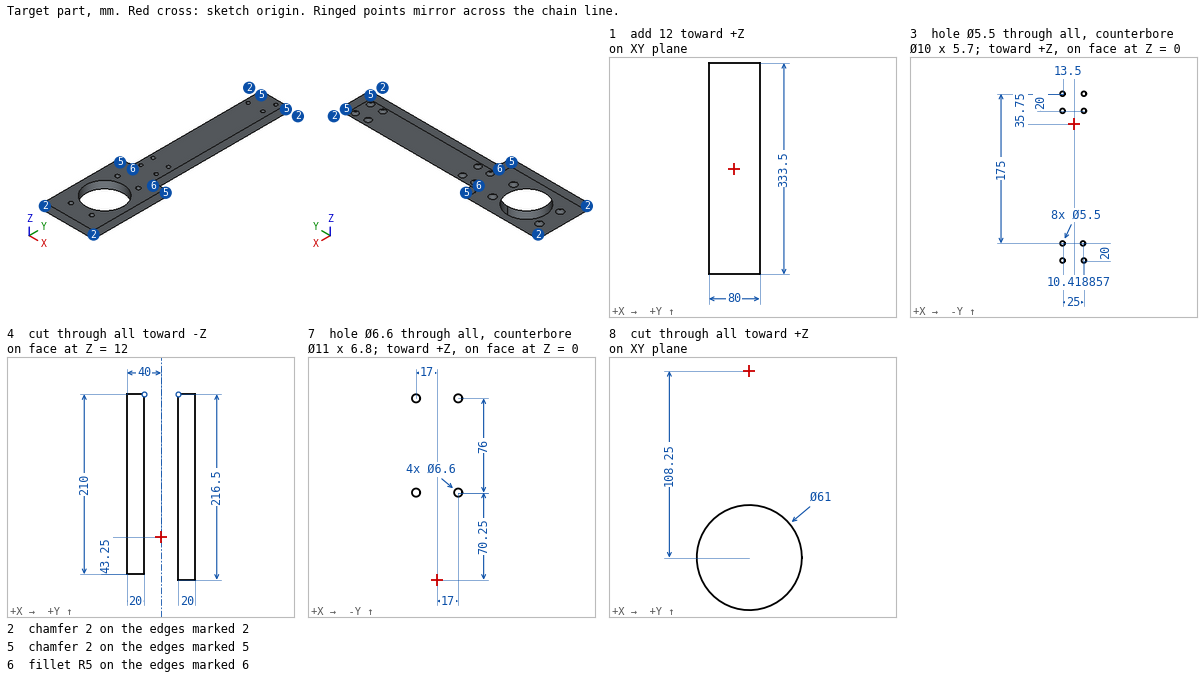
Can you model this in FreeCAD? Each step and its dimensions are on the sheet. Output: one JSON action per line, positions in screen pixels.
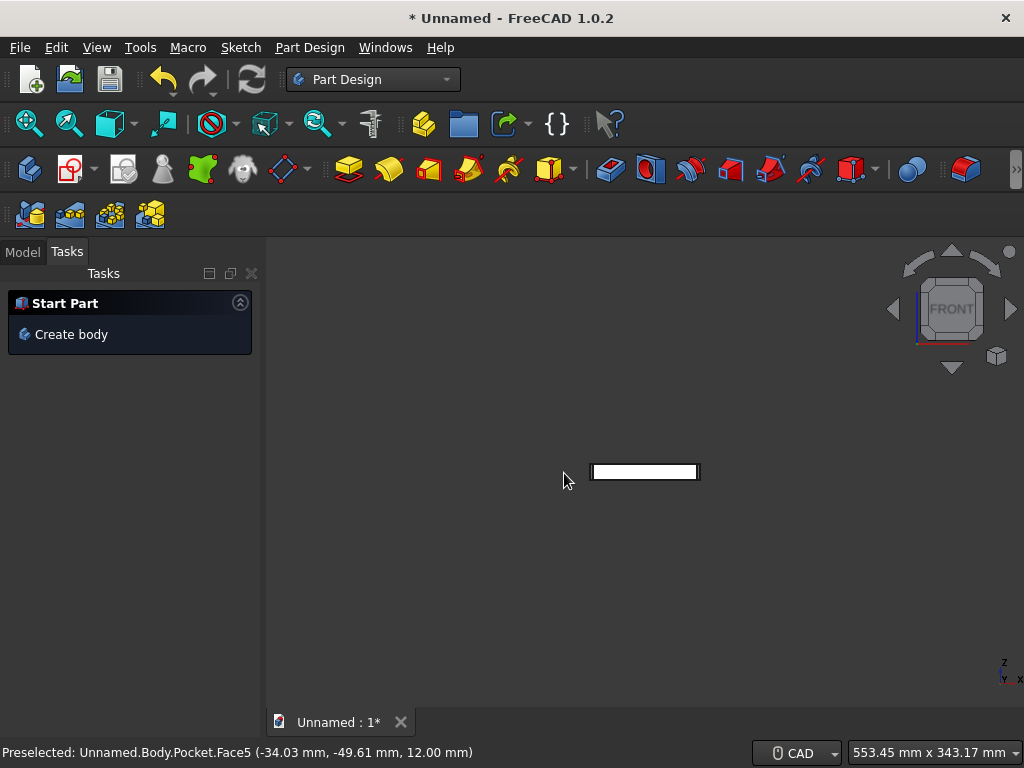
{"action": "key", "text": "v f"}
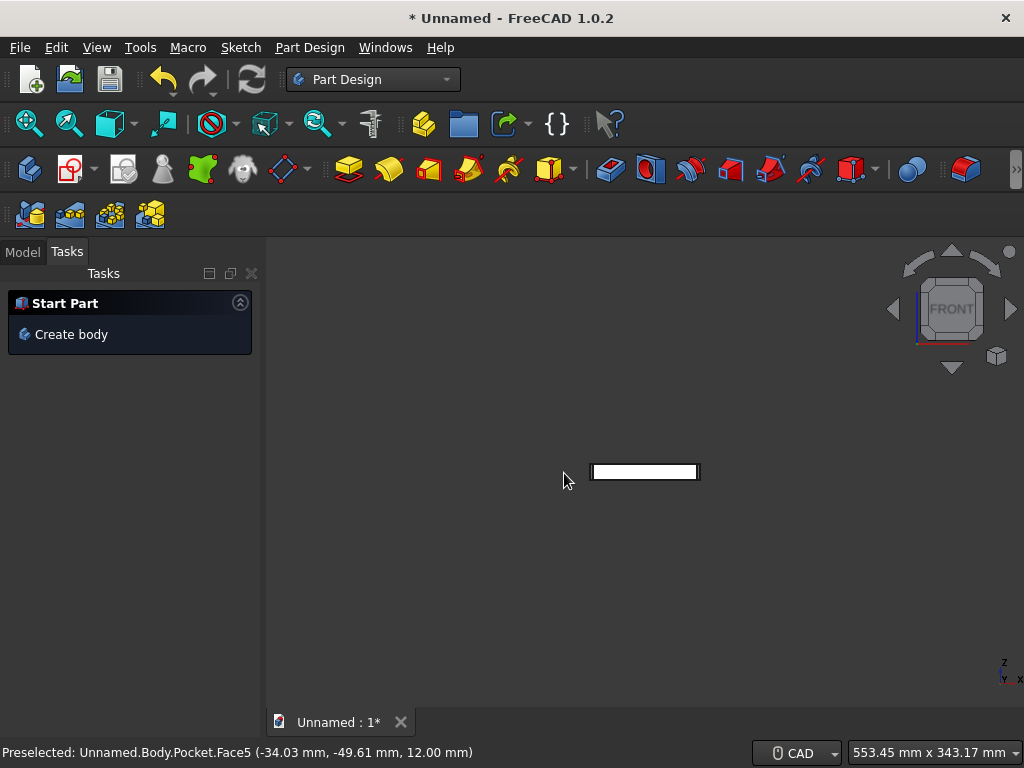
{"action": "scroll", "coordinate": [590, 471], "scroll_direction": "up", "scroll_amount": 5}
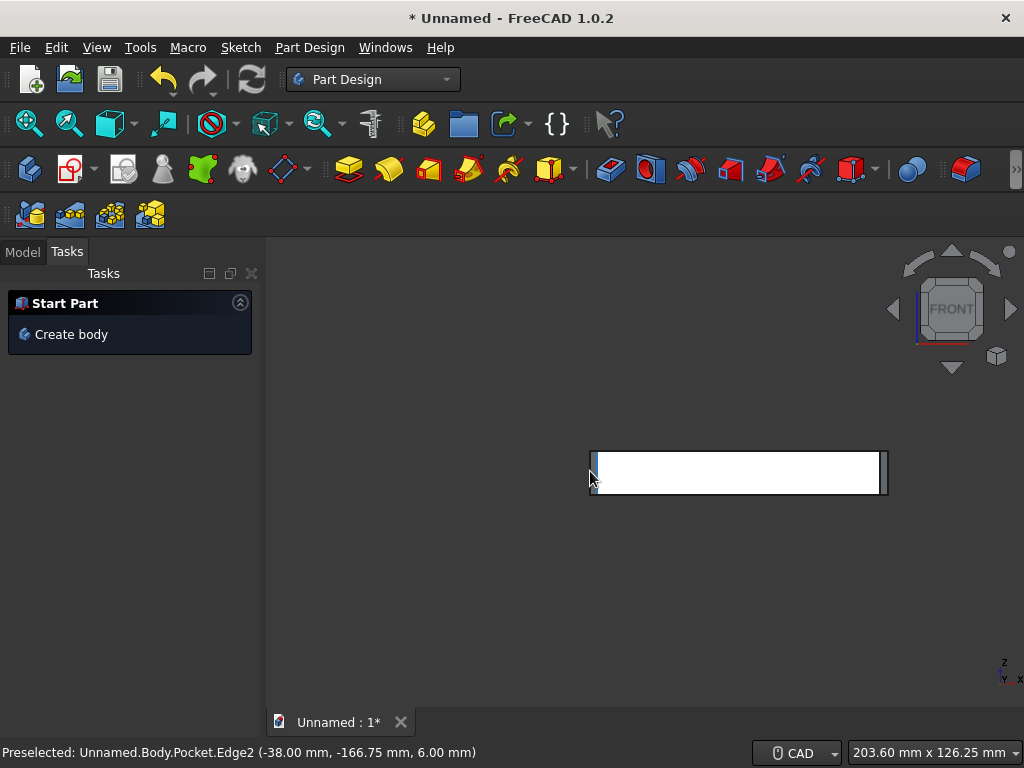
{"action": "key", "text": "v f"}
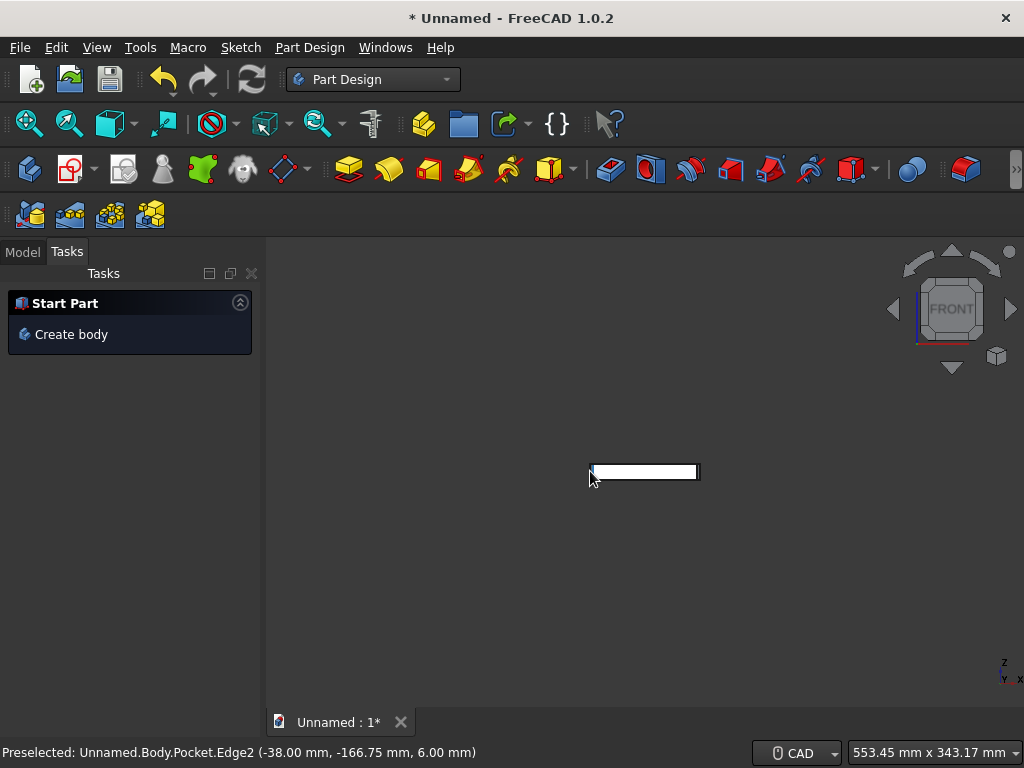
{"action": "key", "text": "3"}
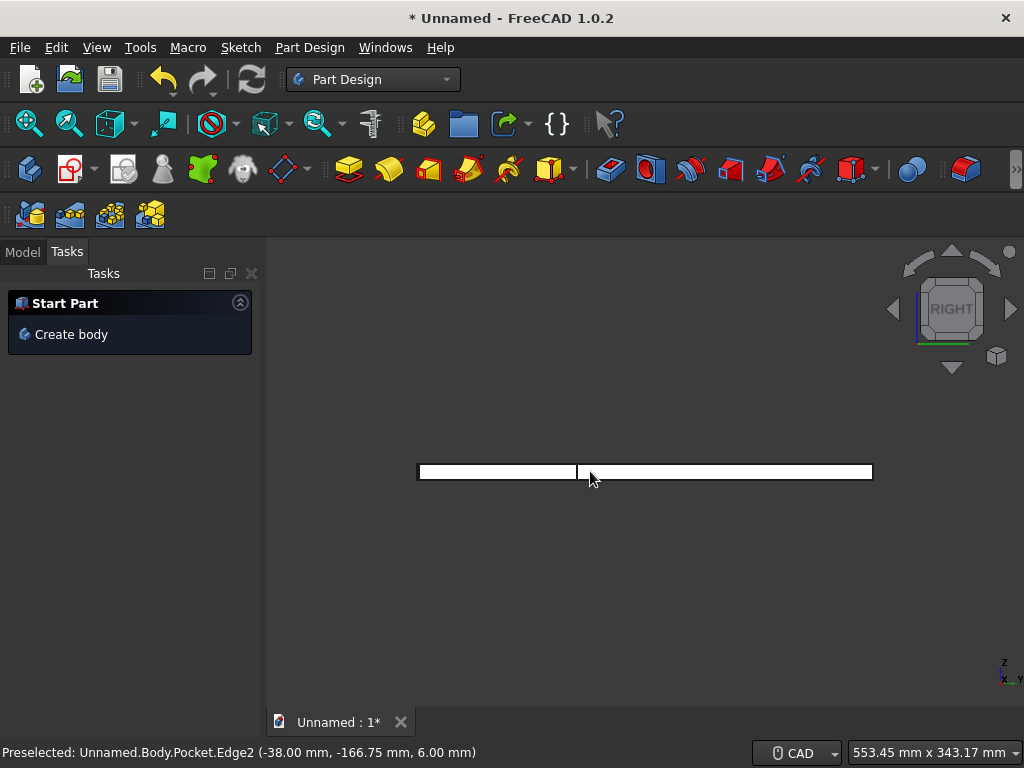
{"action": "left_click", "coordinate": [577, 471]}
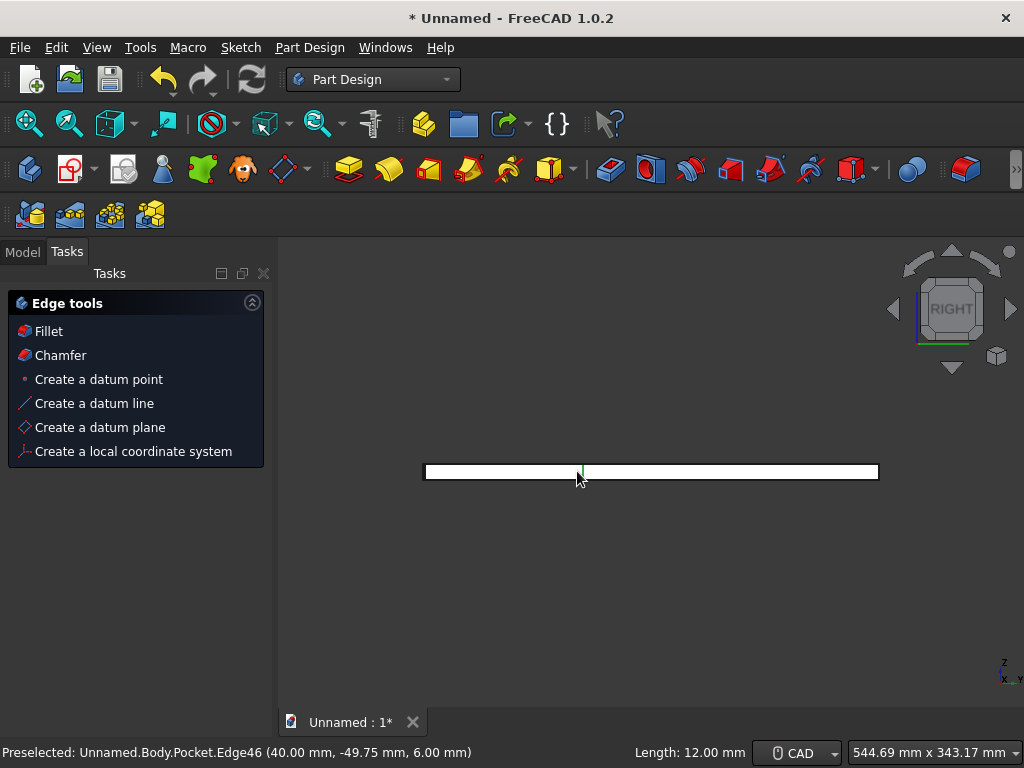
{"action": "left_click", "coordinate": [879, 471], "text": "ctrl"}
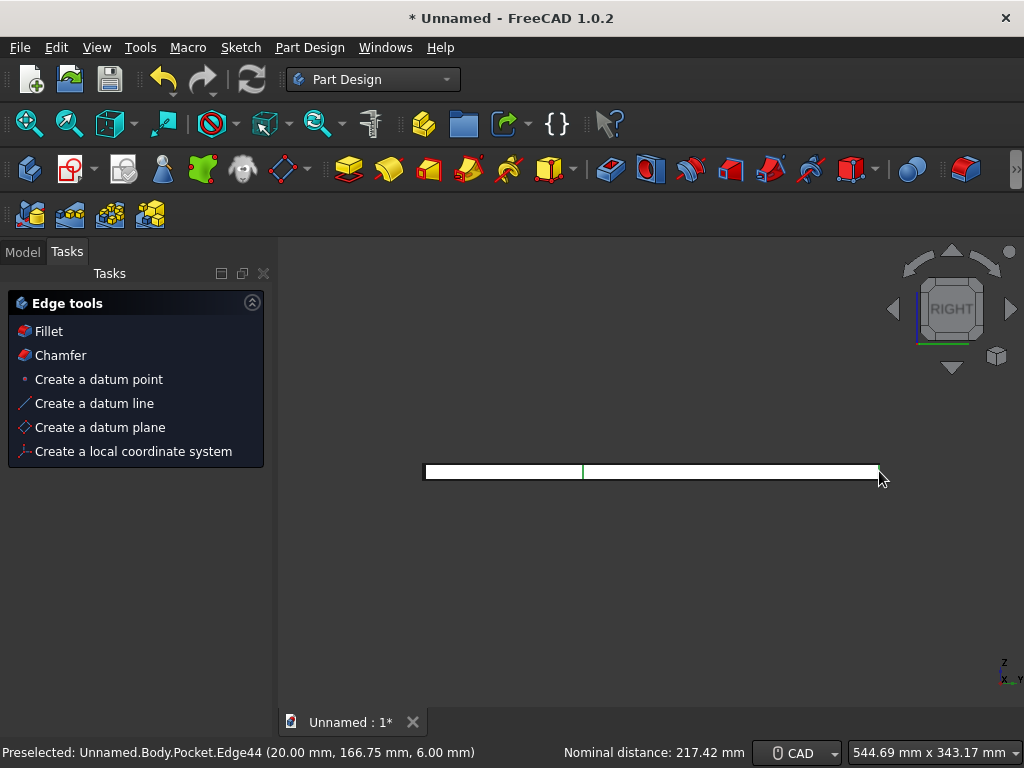
{"action": "scroll", "coordinate": [592, 471], "scroll_direction": "up", "scroll_amount": 5}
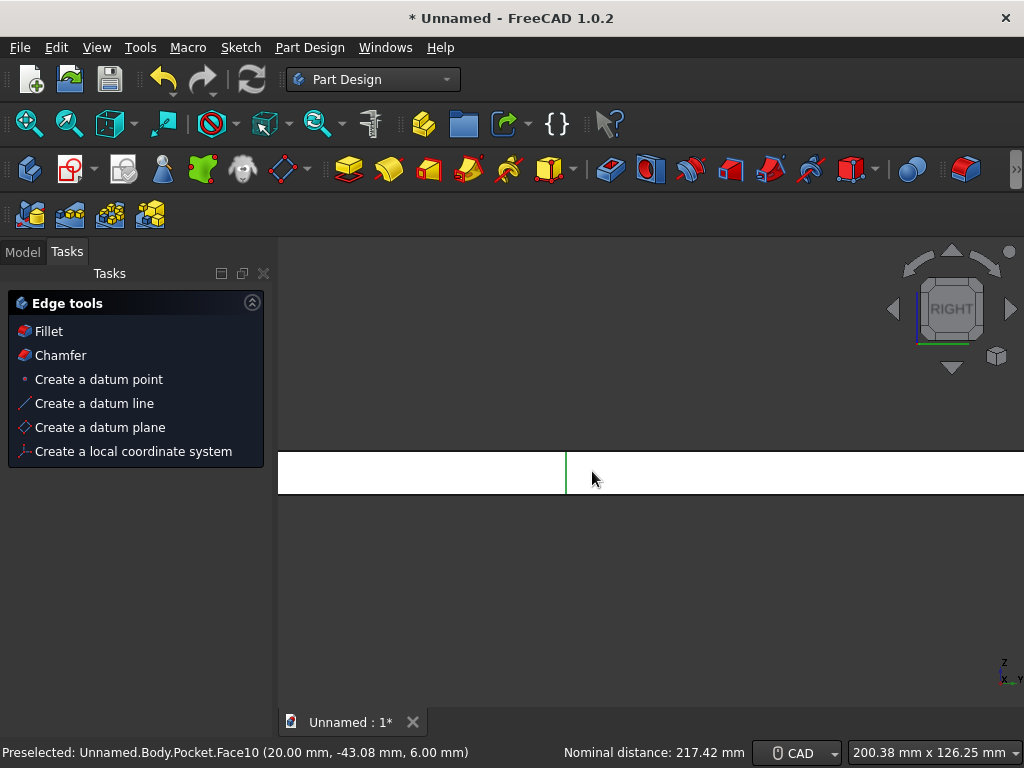
{"action": "left_click", "coordinate": [30, 124]}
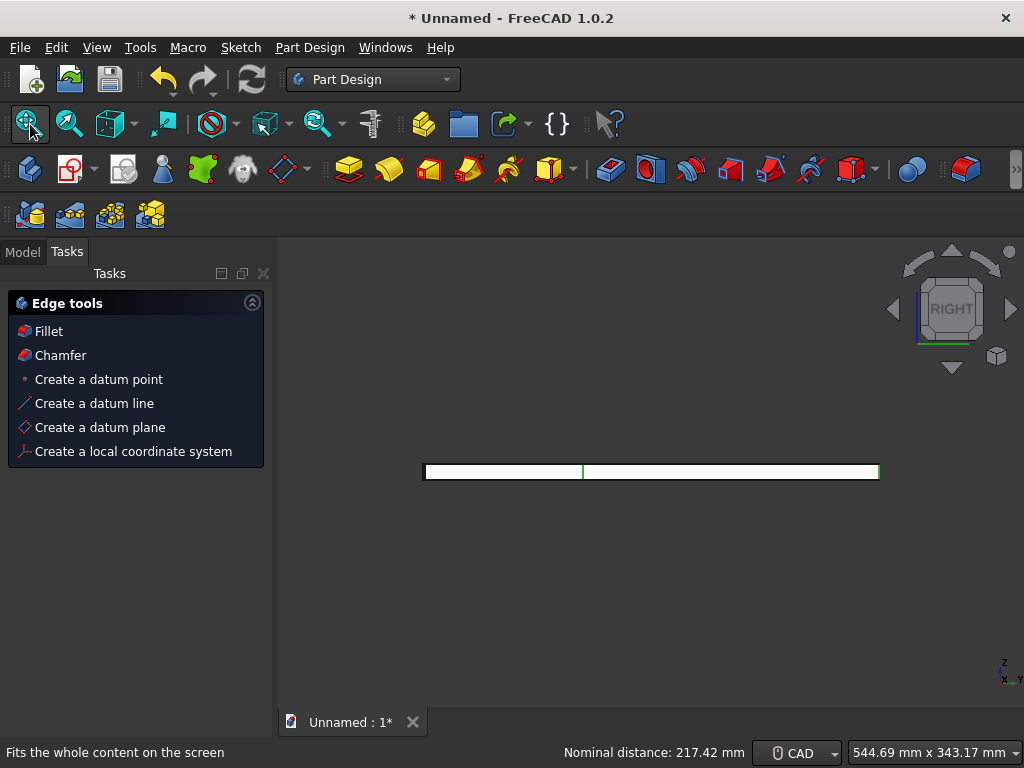
{"action": "key", "text": "5"}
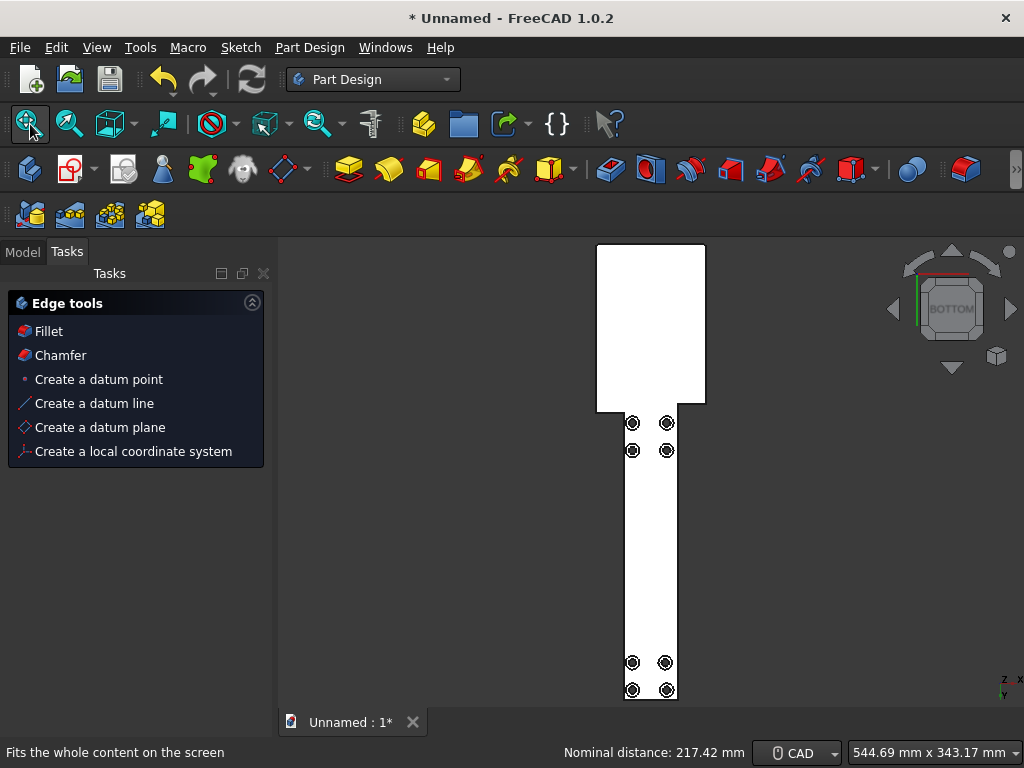
{"action": "scroll", "coordinate": [596, 412], "scroll_direction": "up", "scroll_amount": 5}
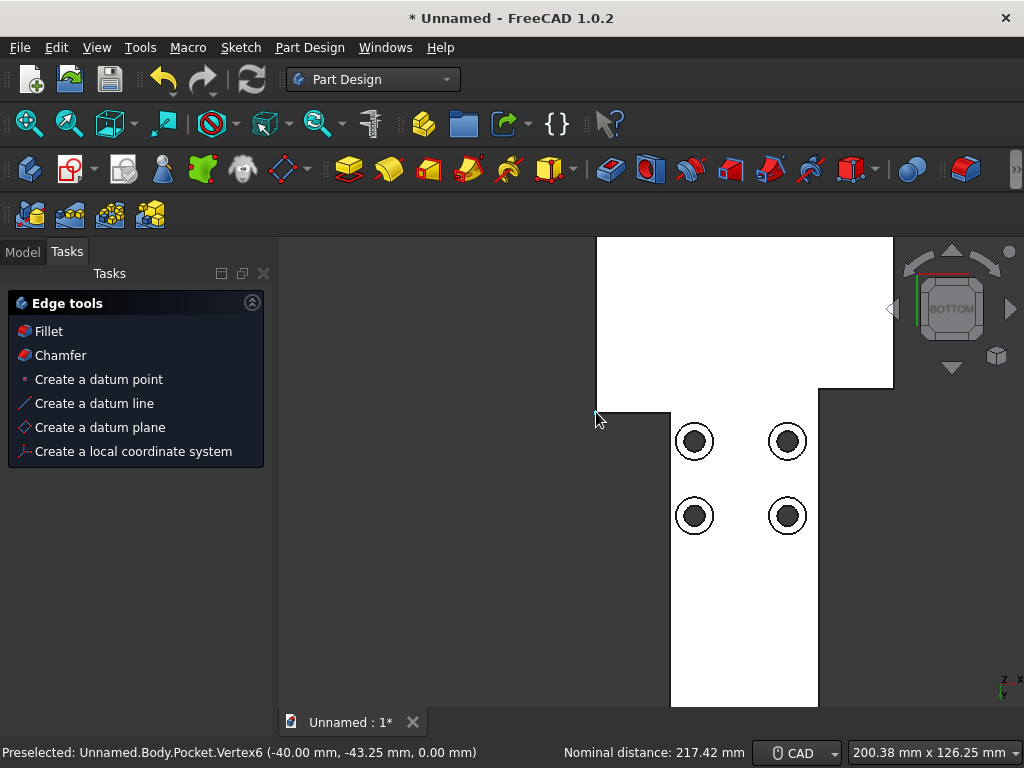
{"action": "key", "text": "v f"}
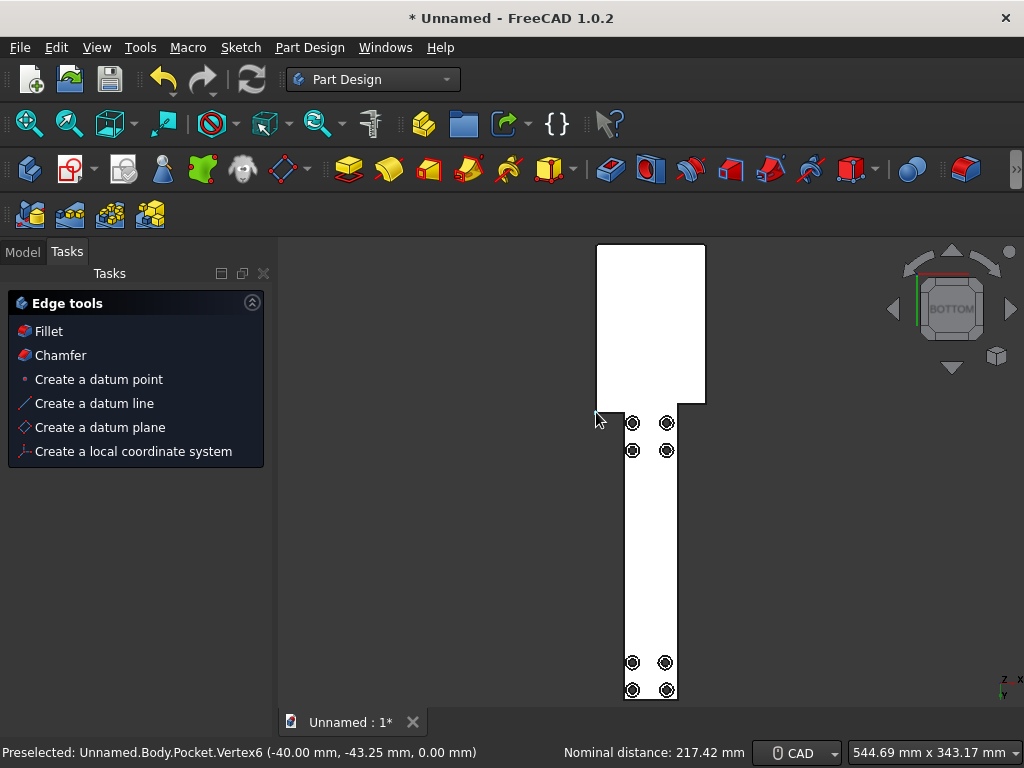
{"action": "key", "text": "4"}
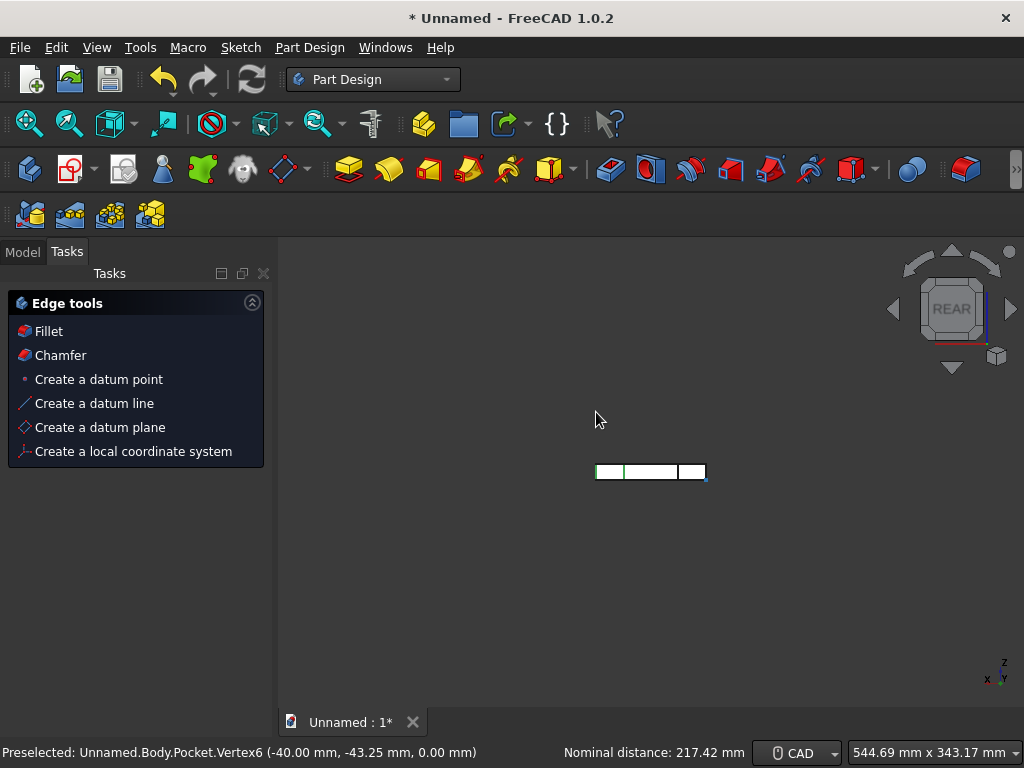
{"action": "key", "text": "v f"}